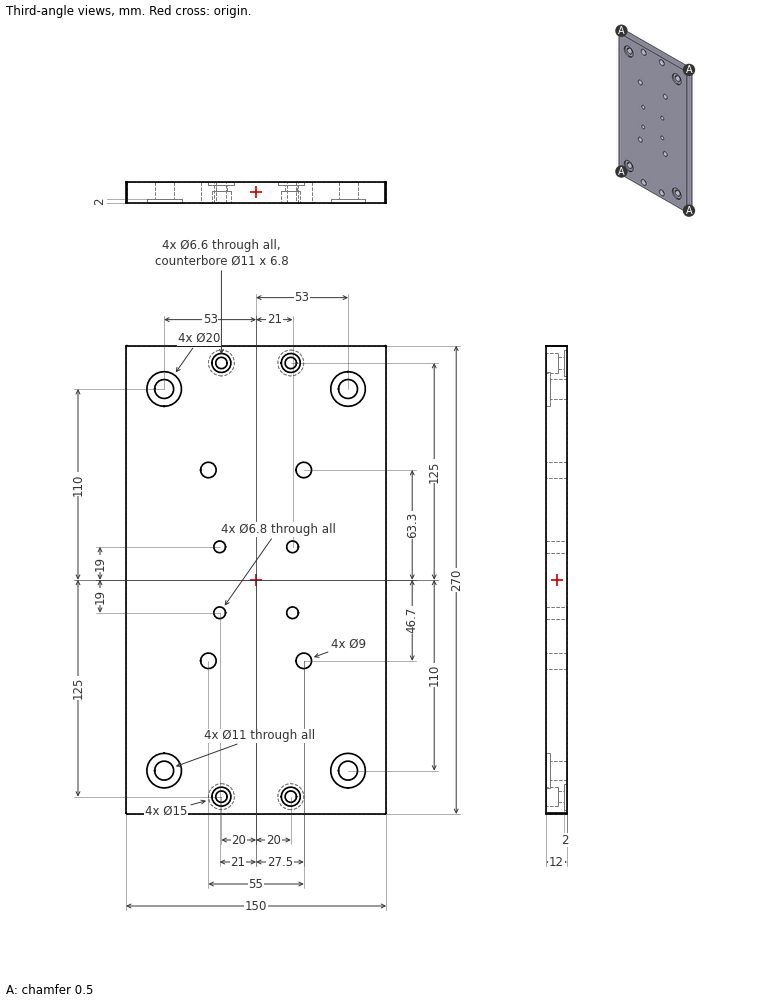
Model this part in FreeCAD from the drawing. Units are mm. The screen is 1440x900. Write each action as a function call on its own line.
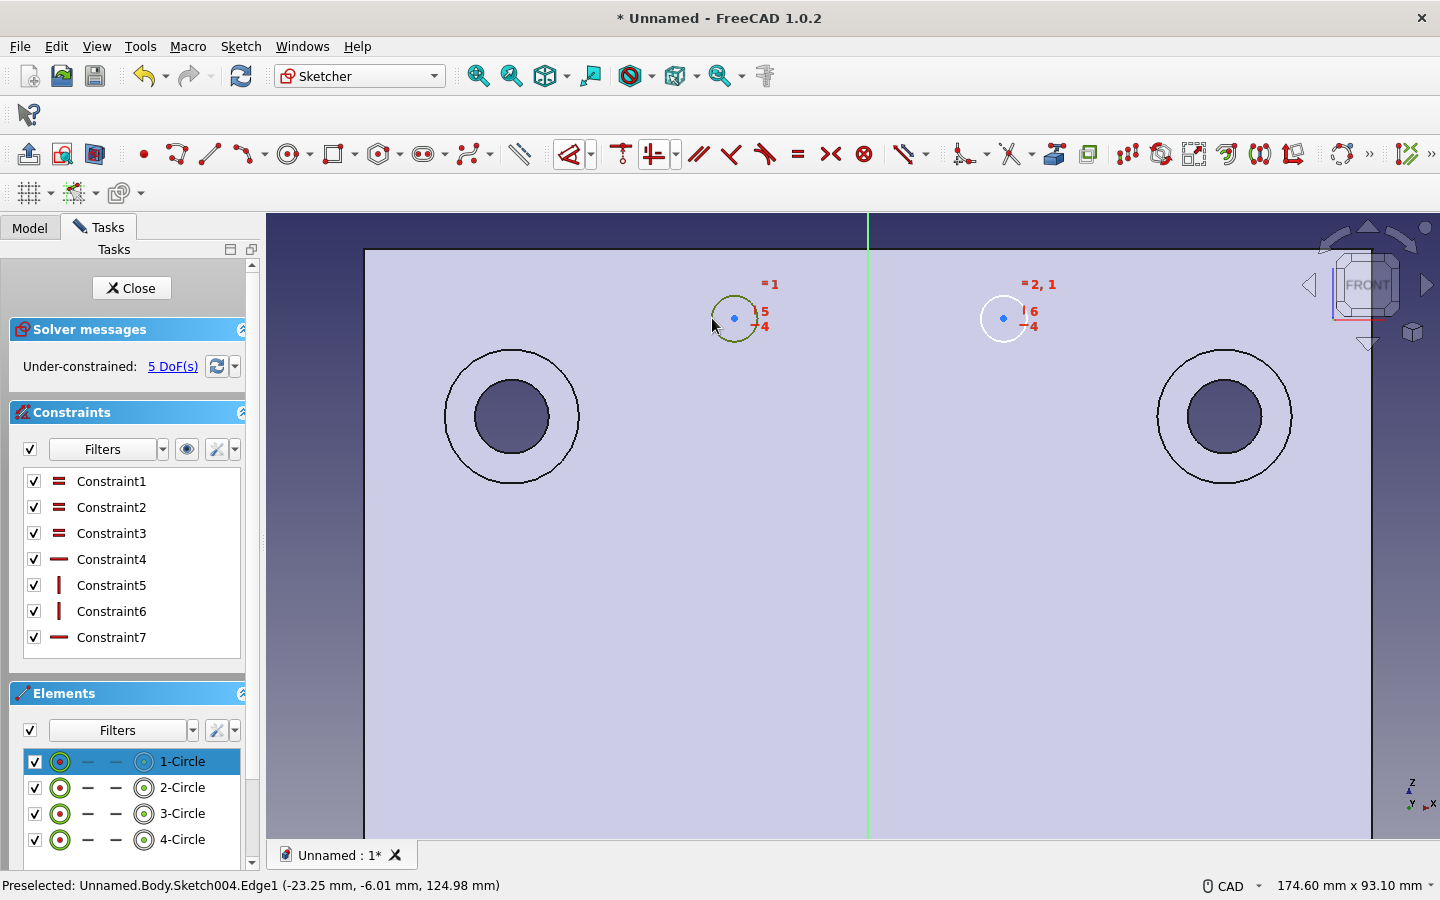
key(k)
key(o)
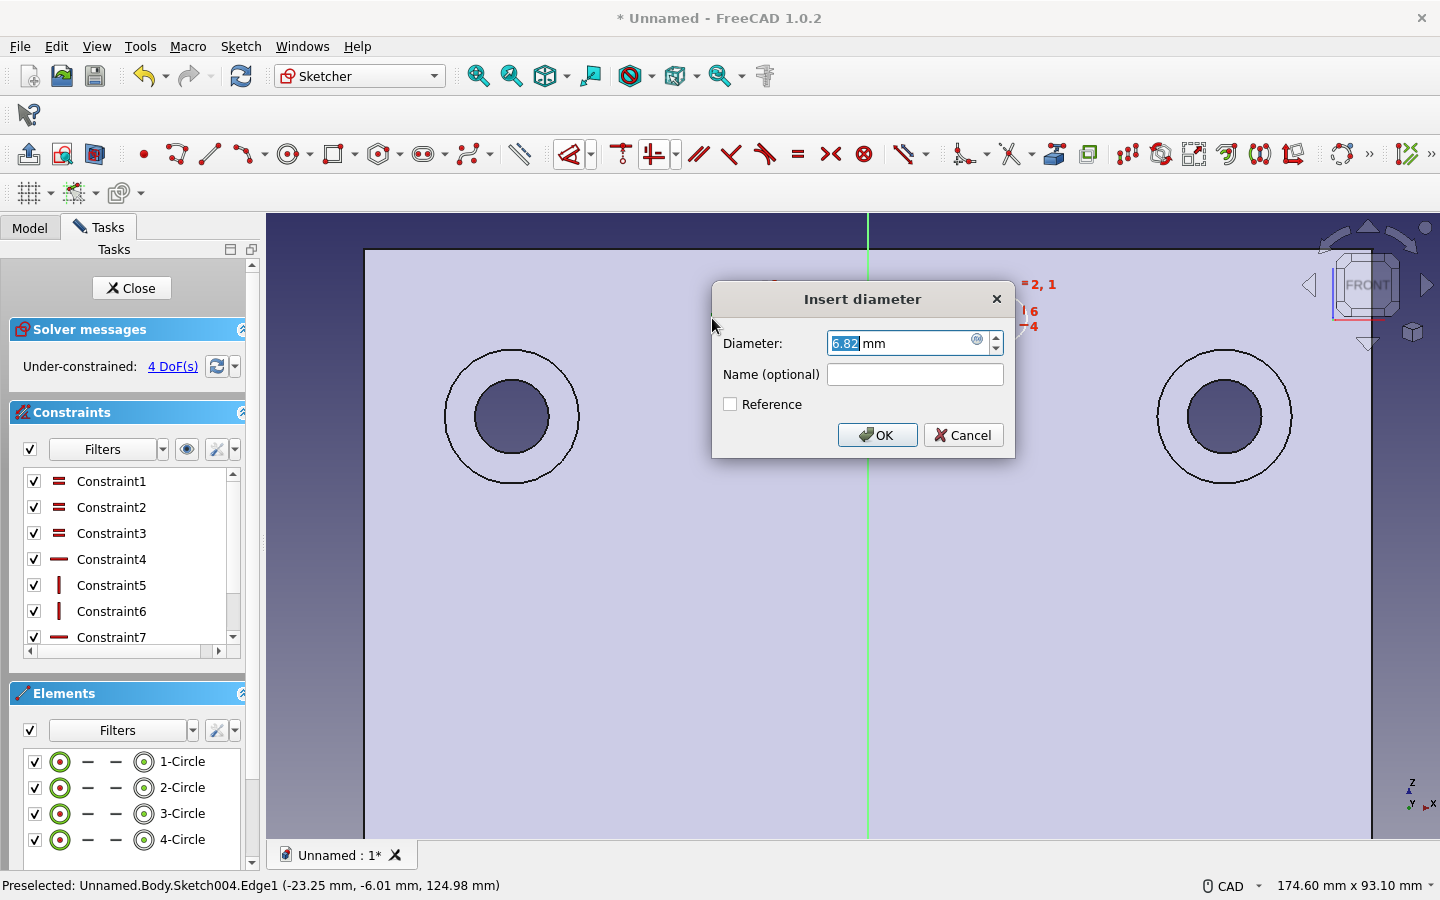
text(6.6)
key(Return)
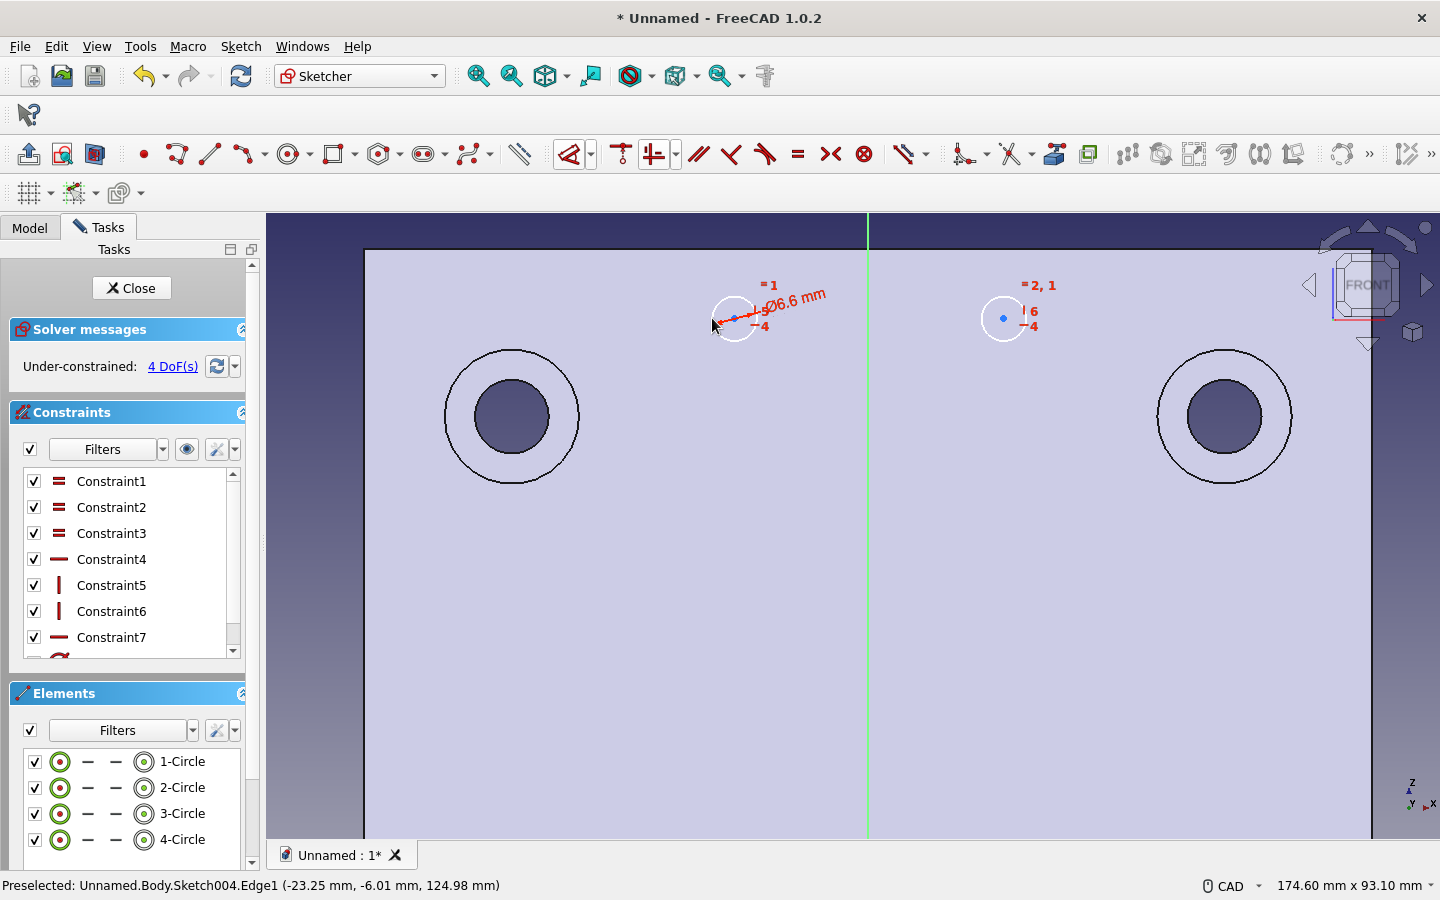
click(735, 319)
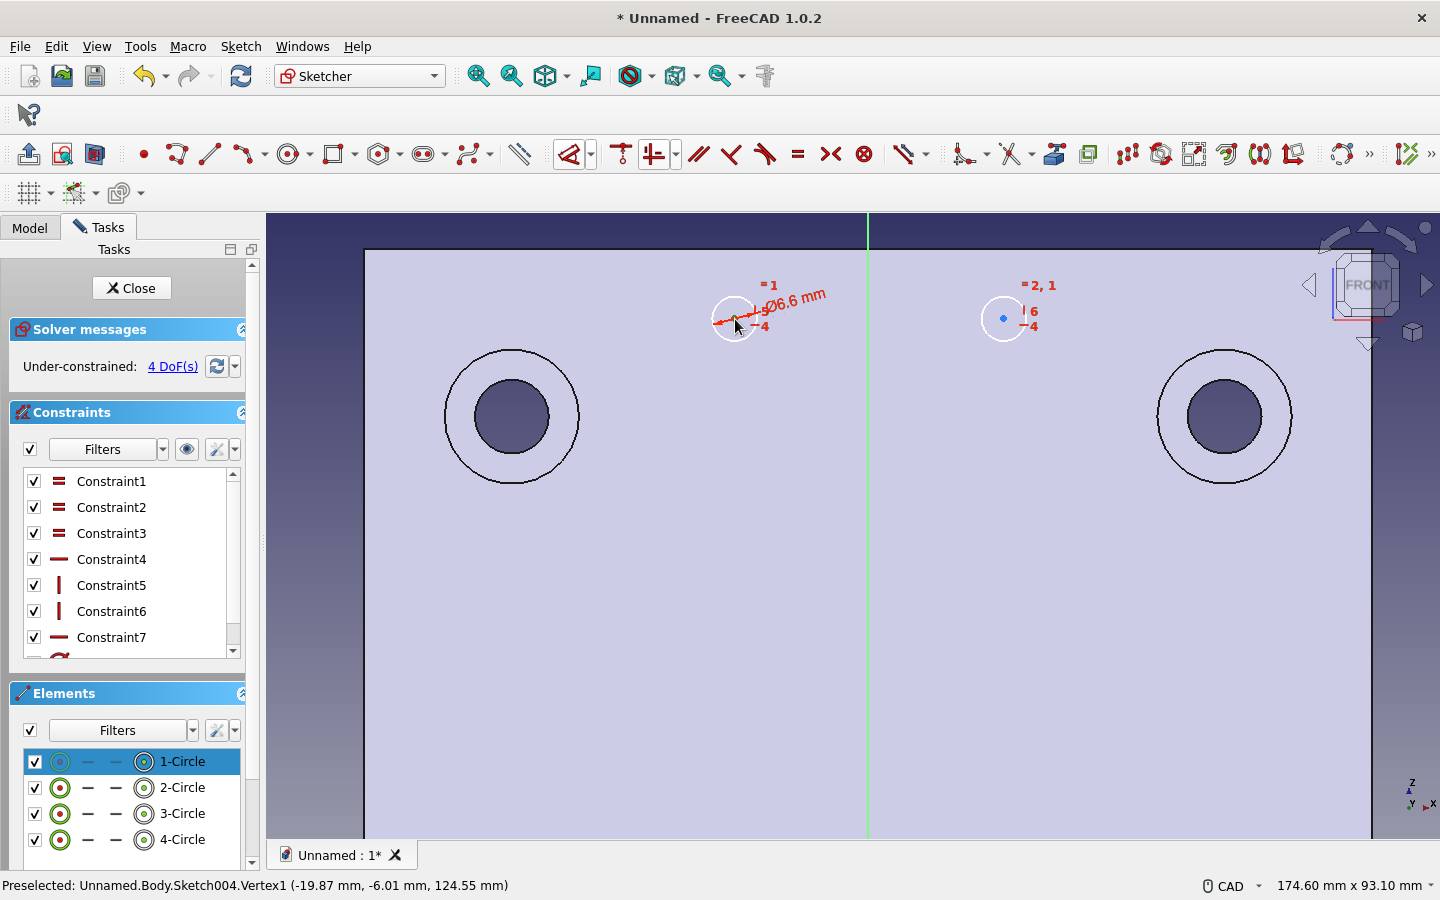
click(590, 154)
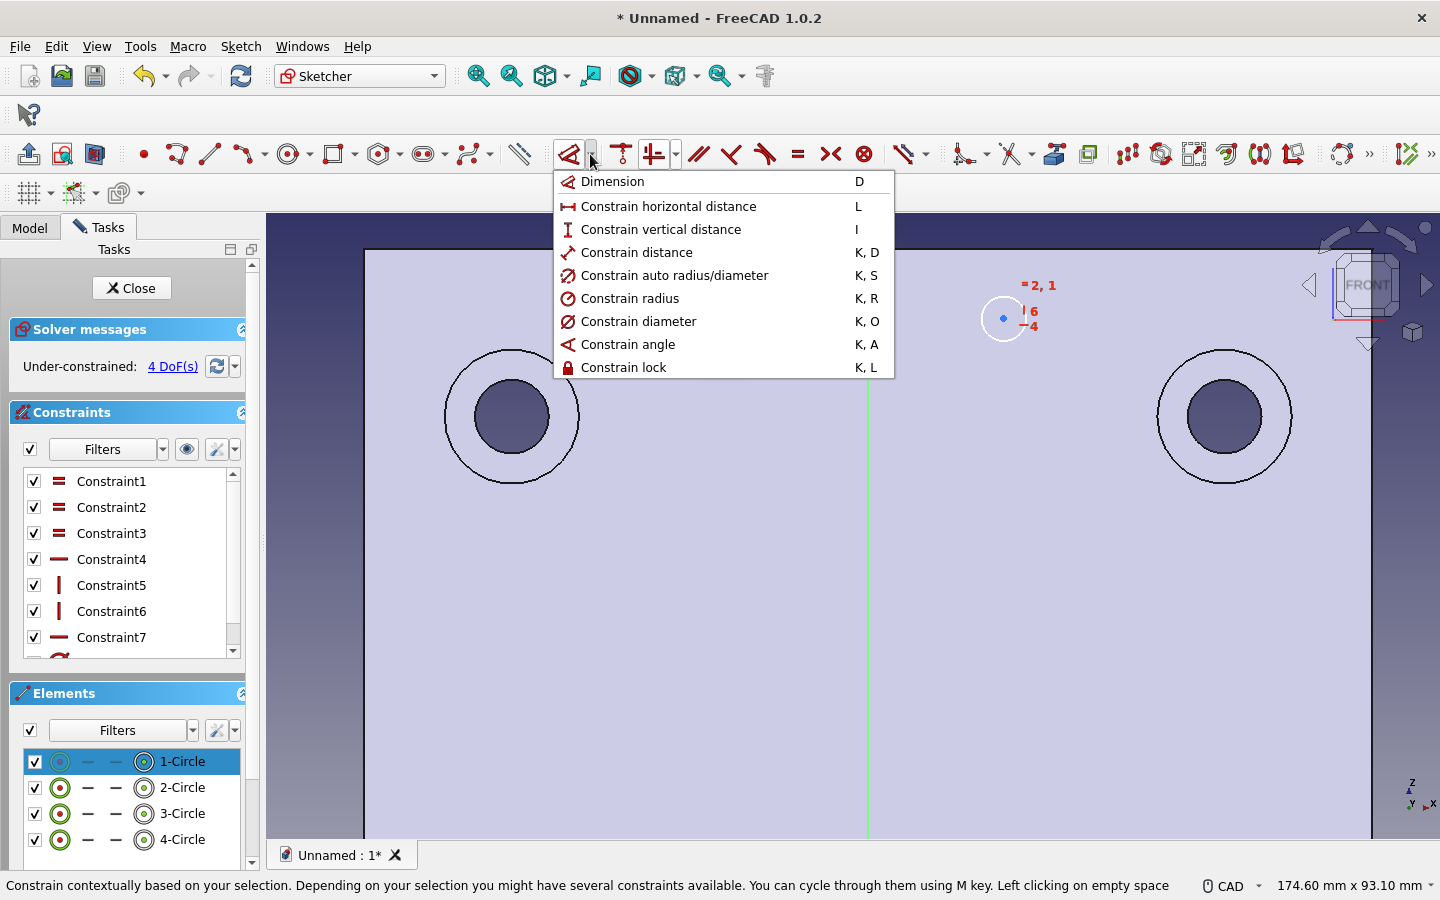
click(724, 206)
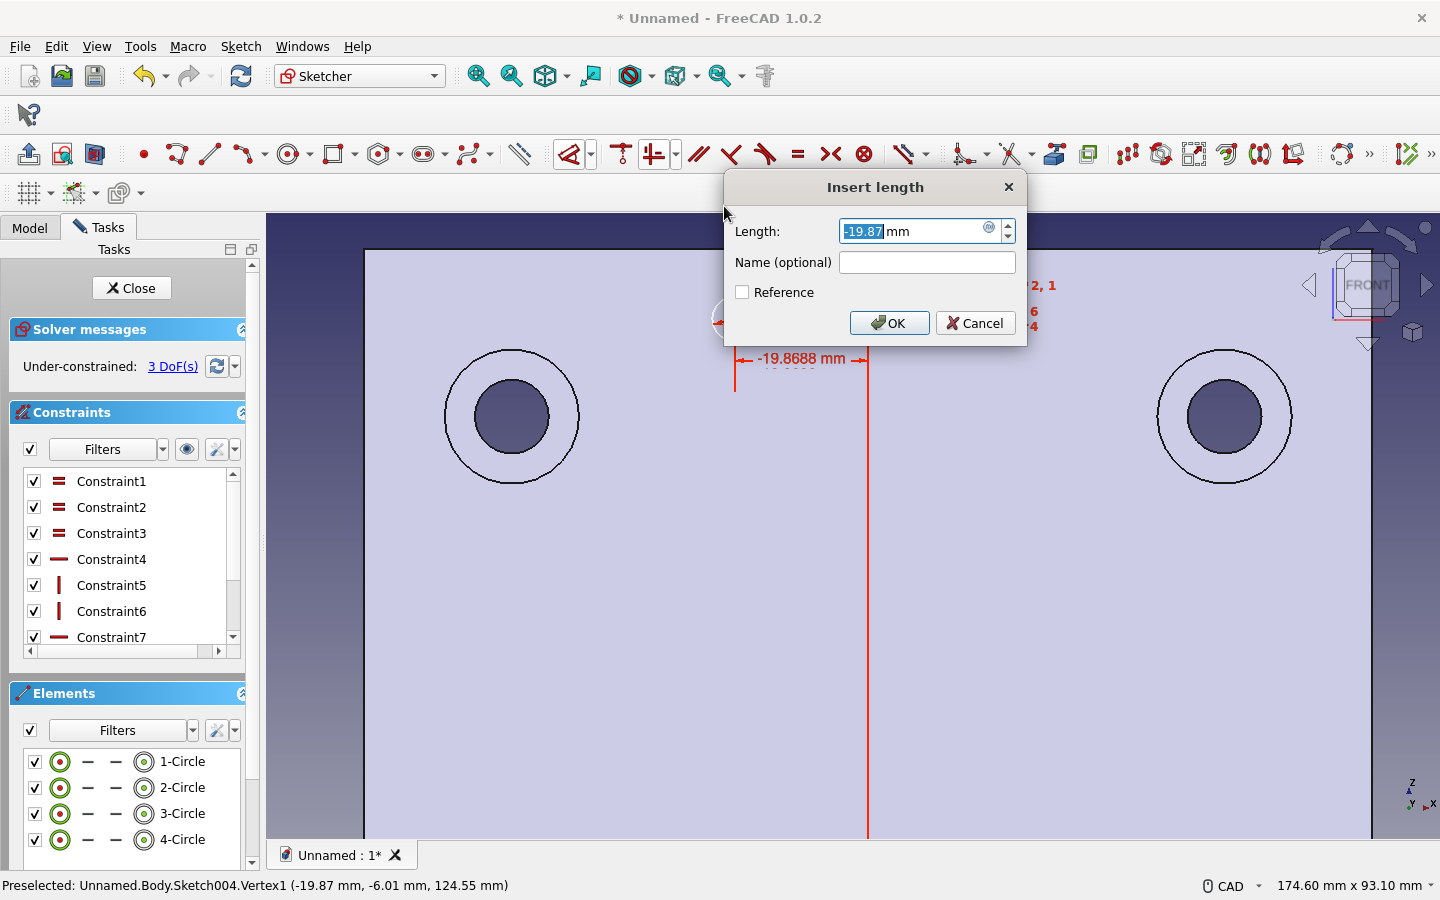
text(-20)
key(Return)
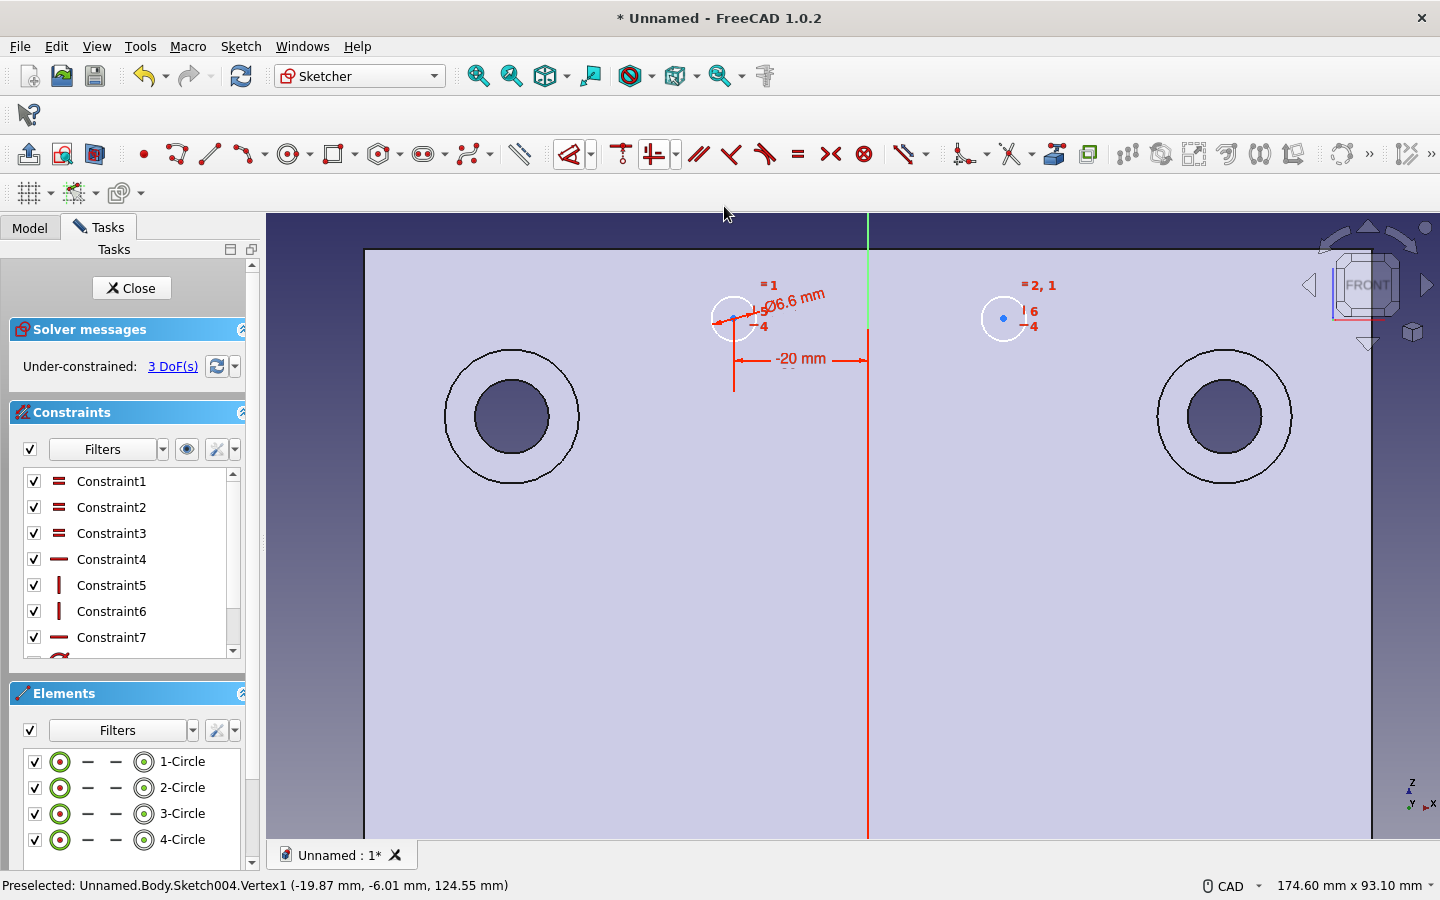
click(1004, 319)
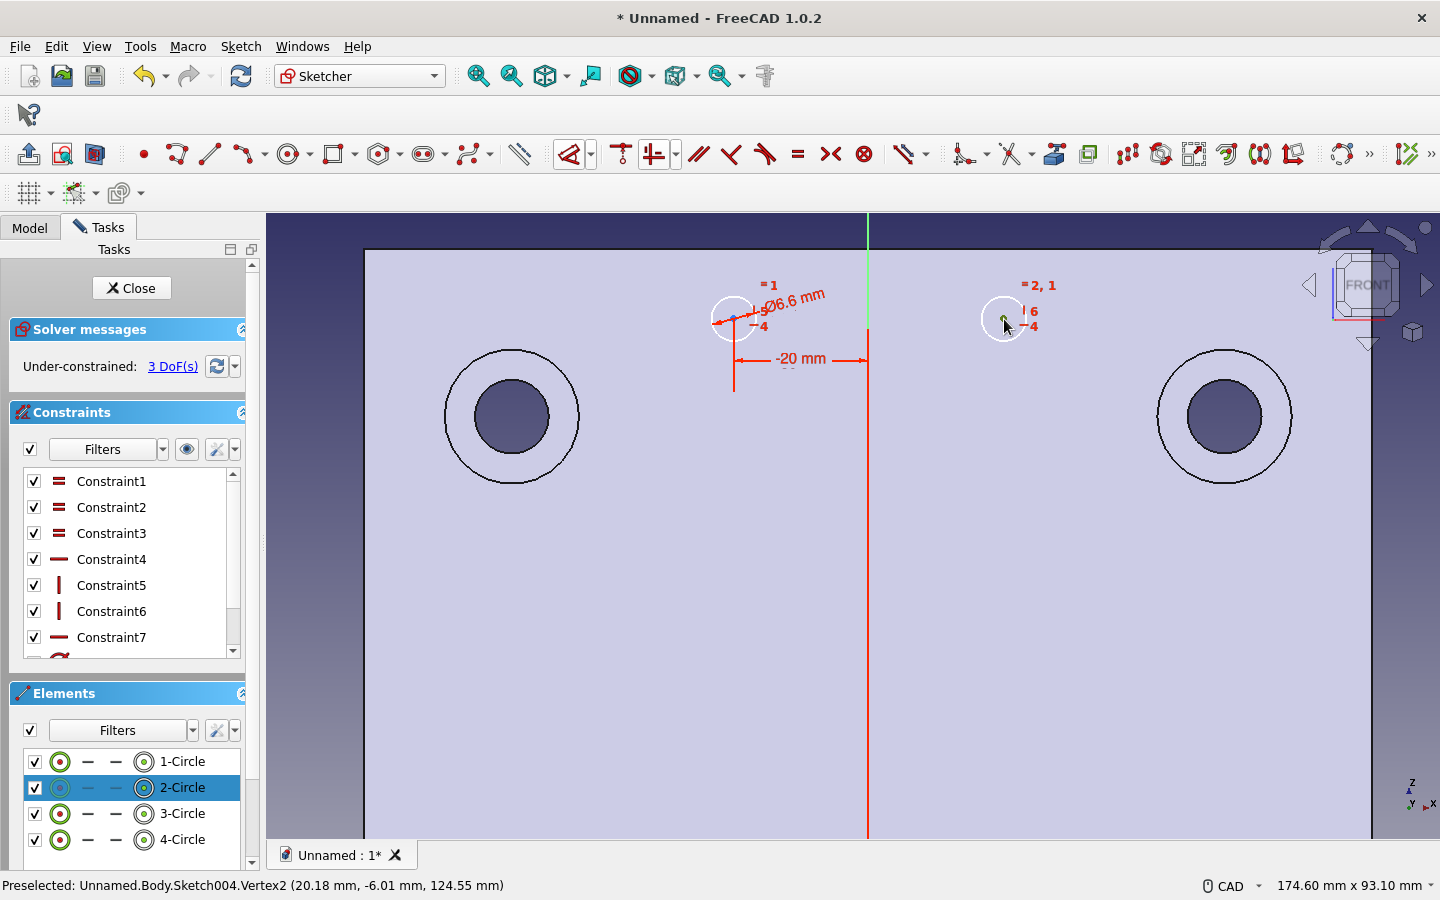
key(l)